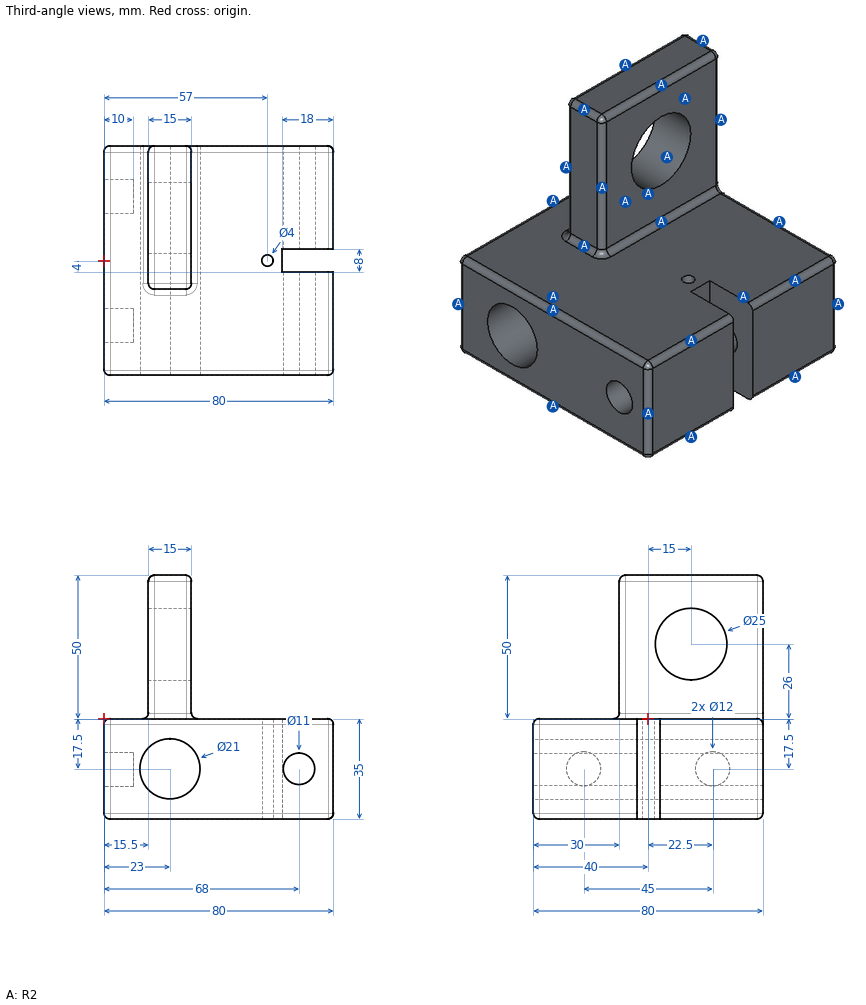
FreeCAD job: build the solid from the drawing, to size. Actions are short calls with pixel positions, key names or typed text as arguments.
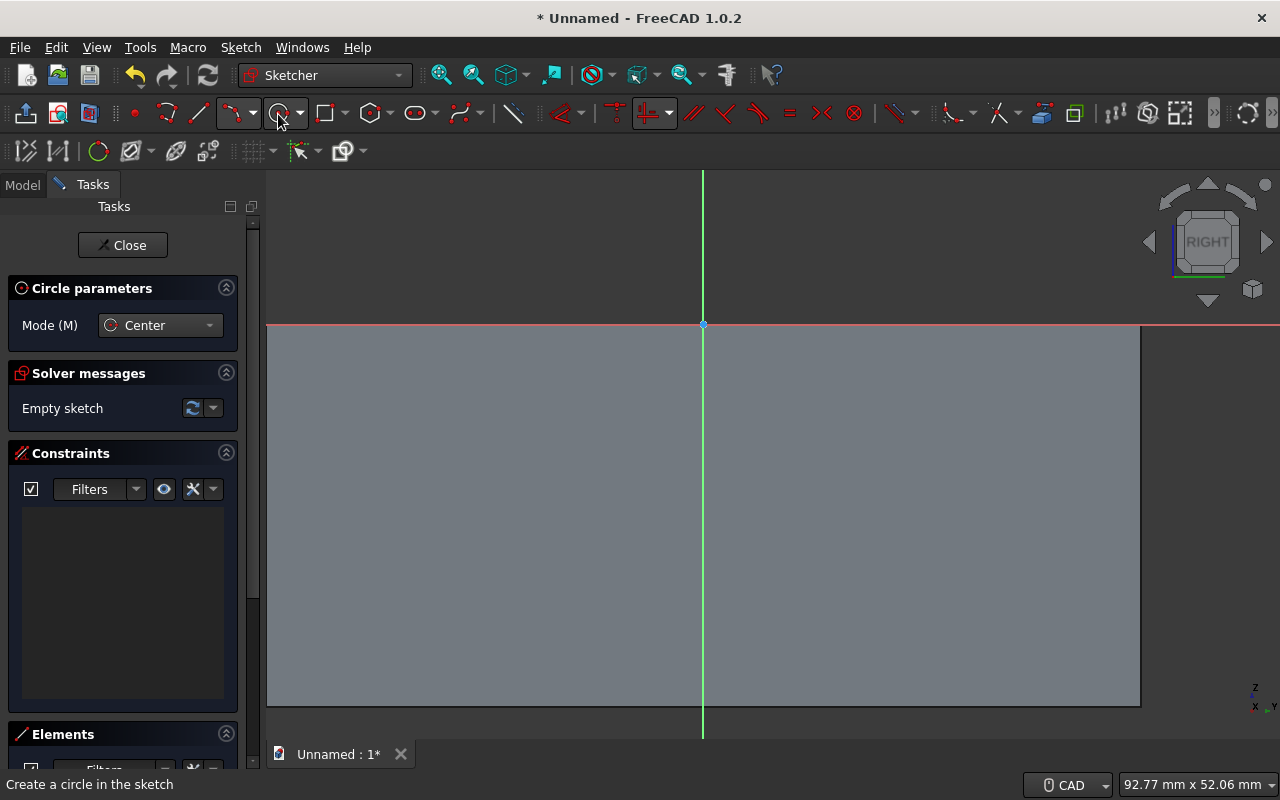
click(949, 516)
click(996, 470)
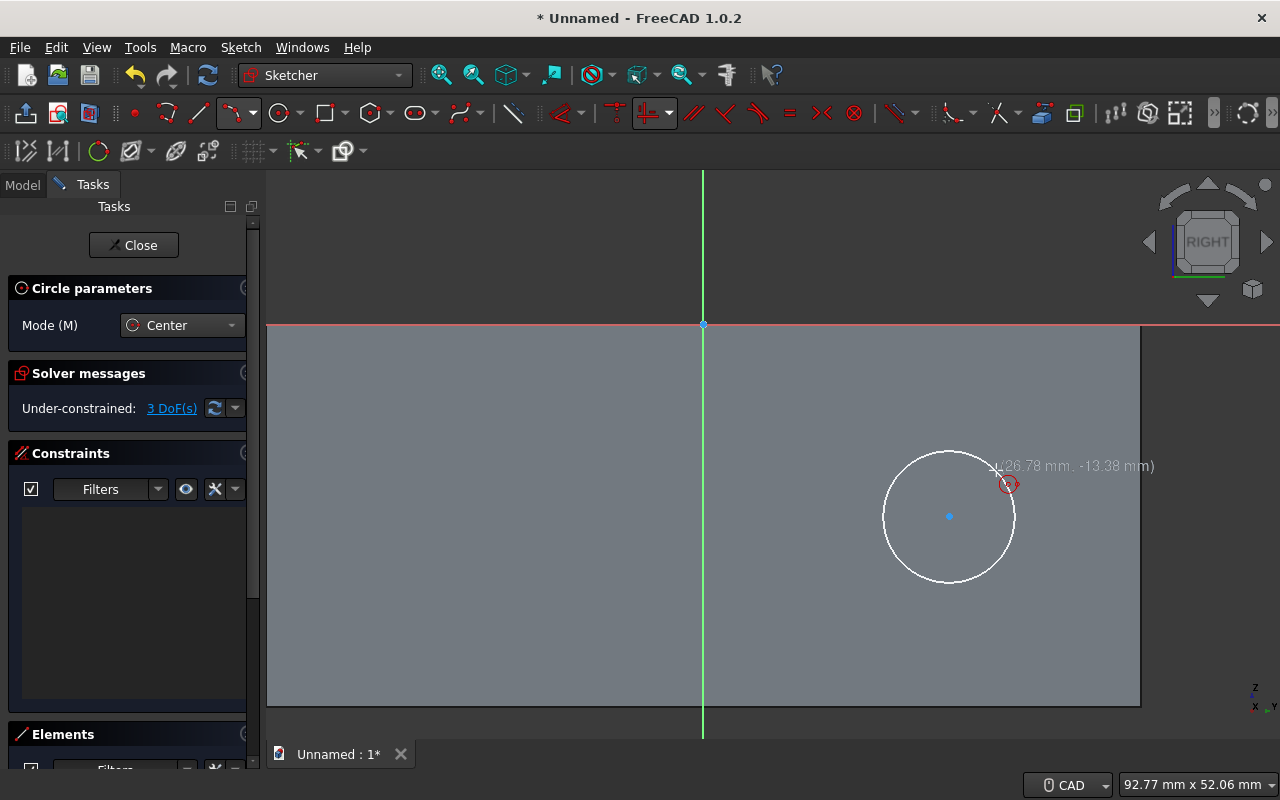
click(457, 516)
click(504, 470)
key(Escape)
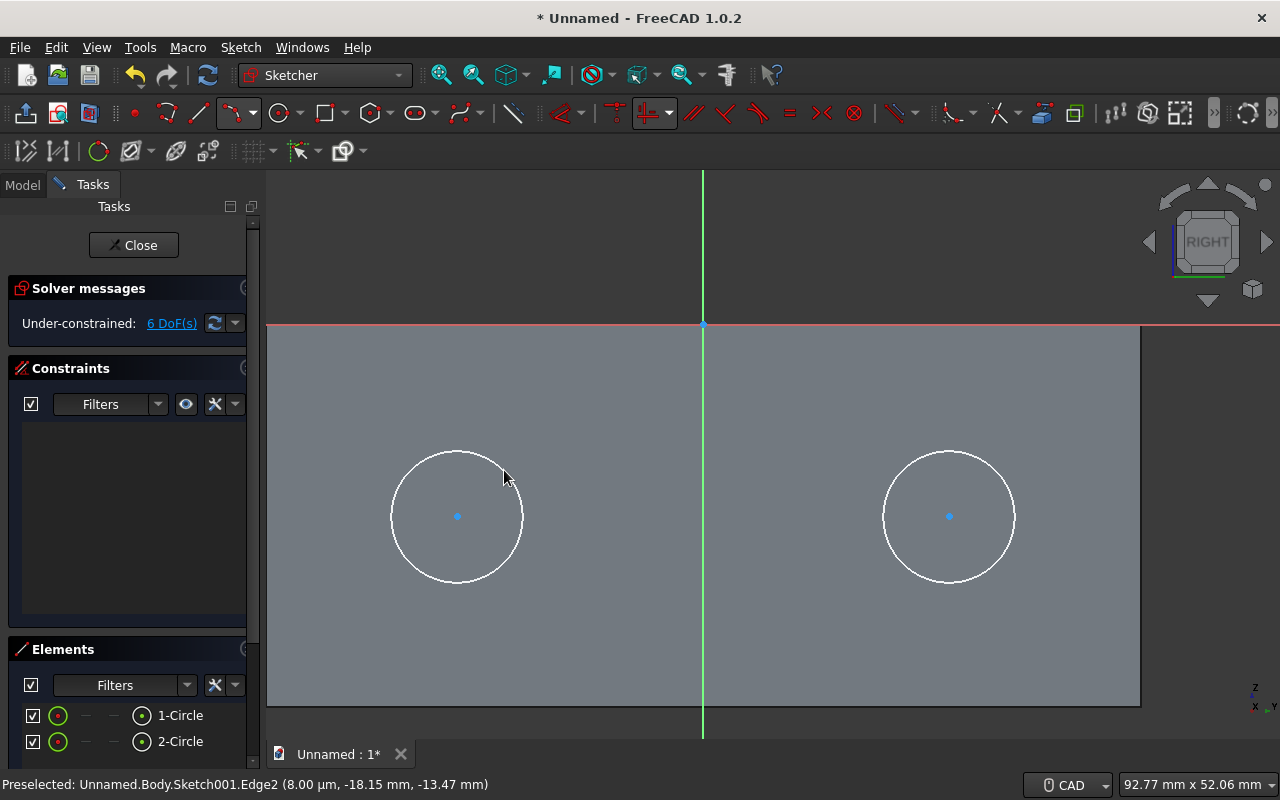
click(995, 470)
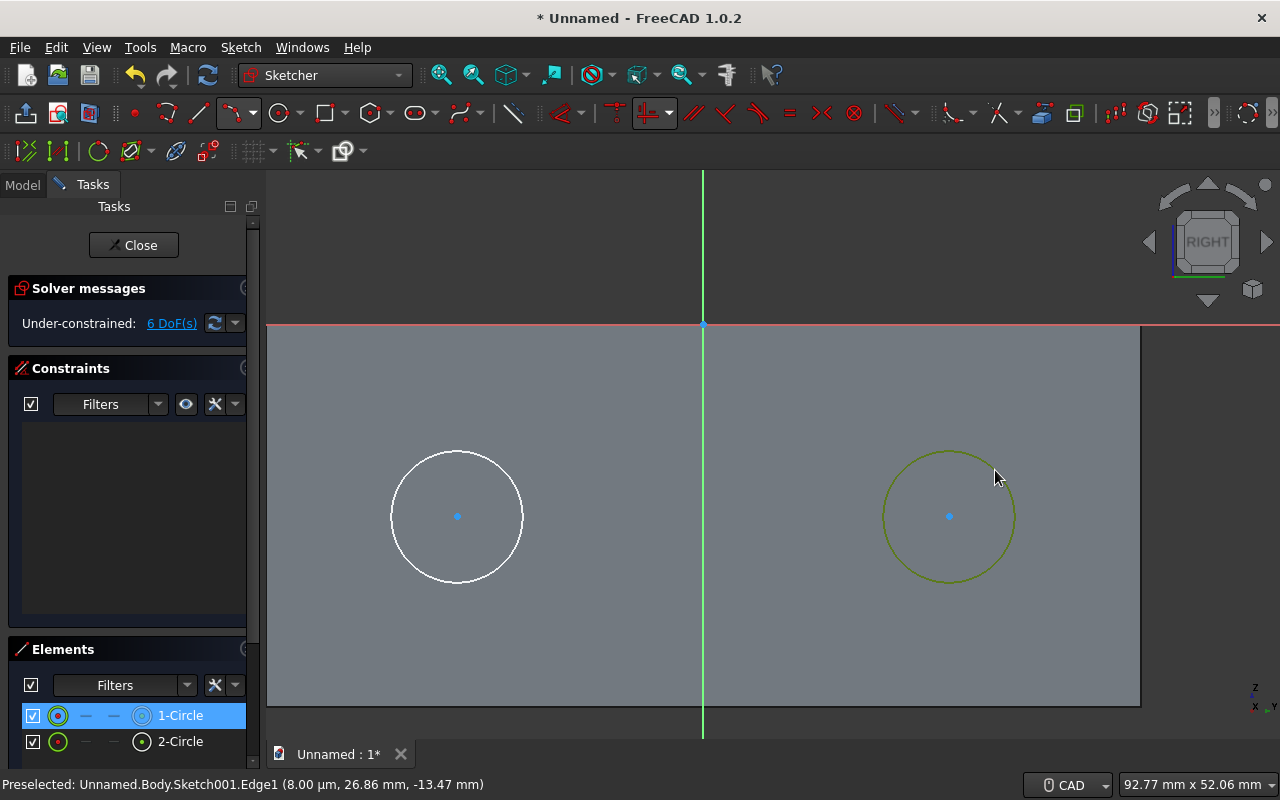
click(503, 470)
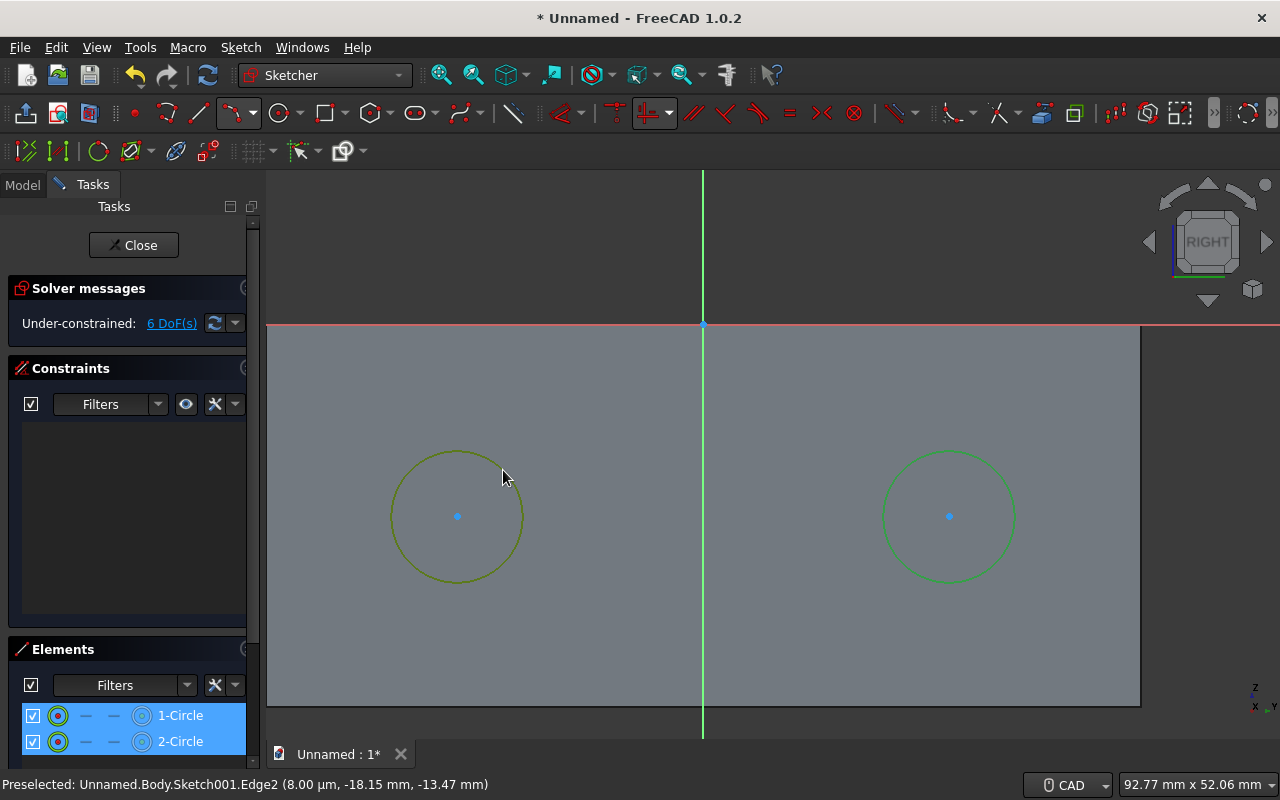
click(790, 114)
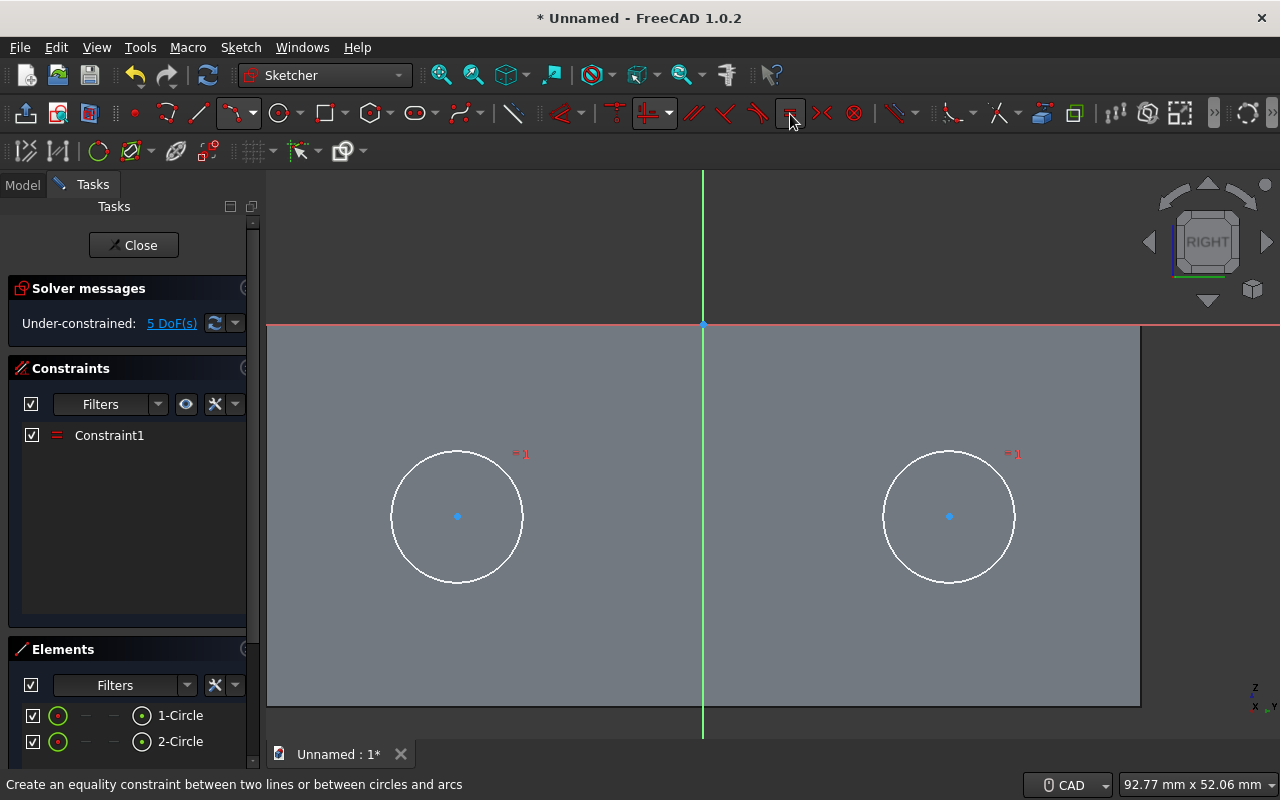
click(949, 517)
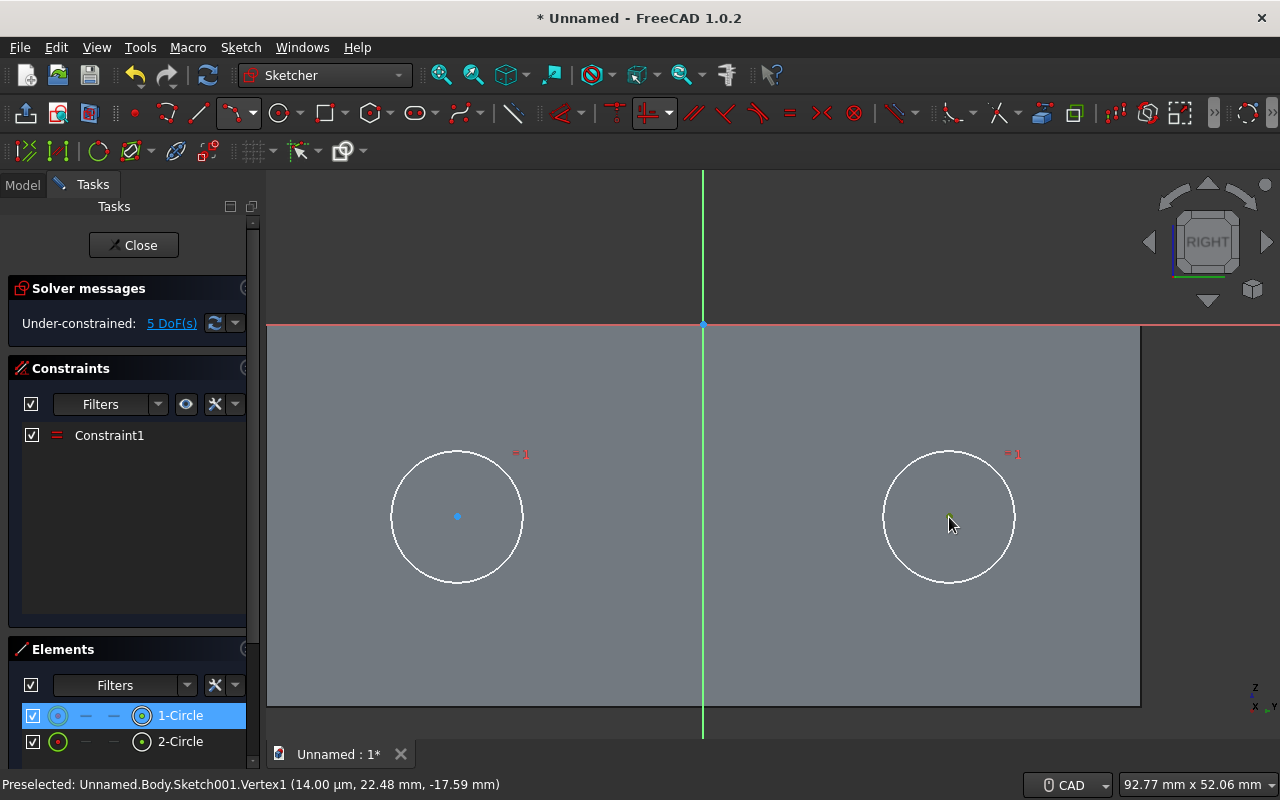
click(457, 517)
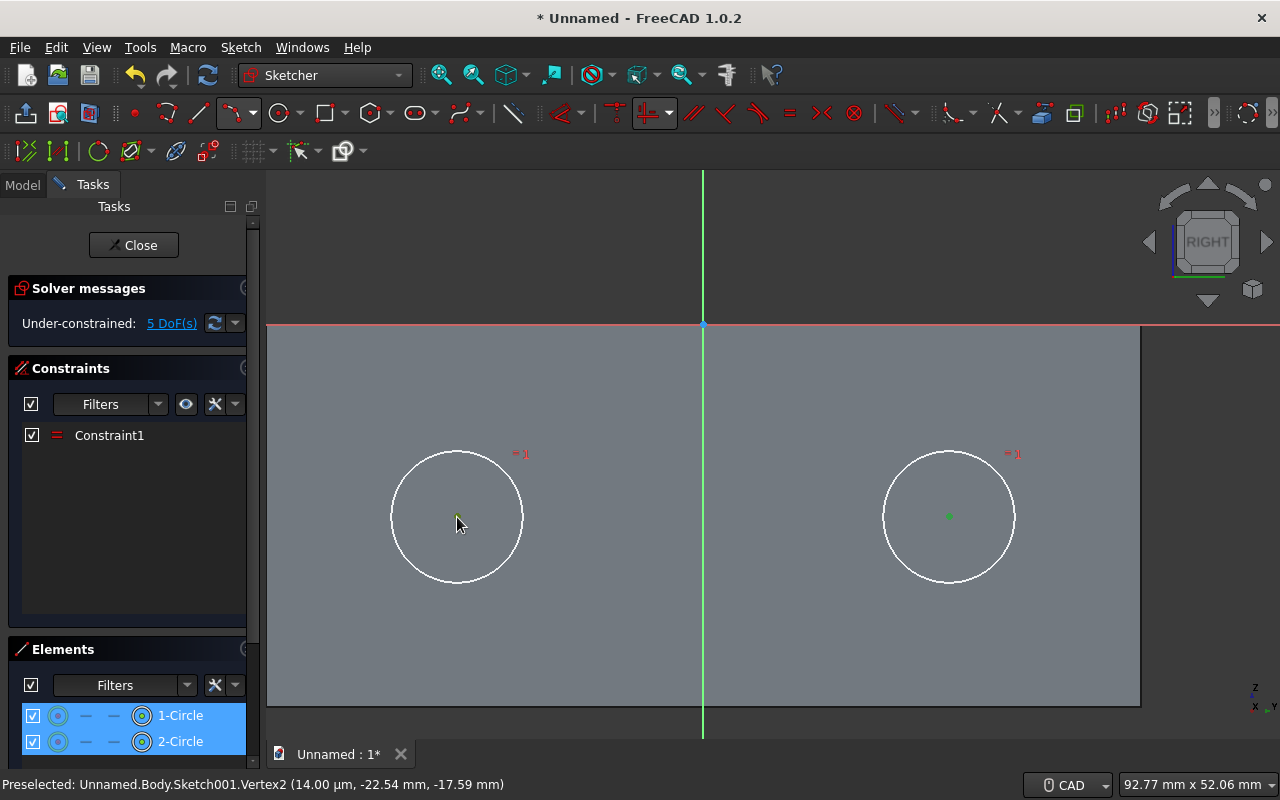
key(h)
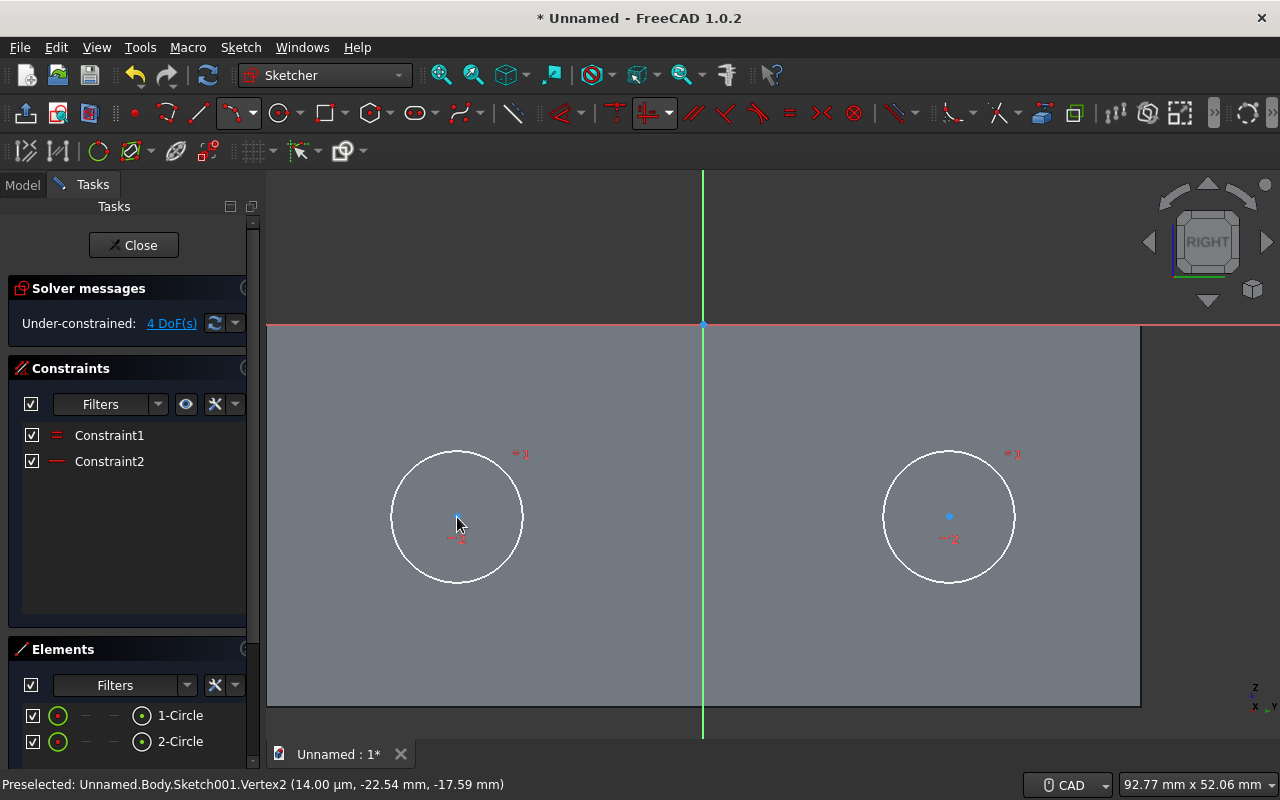
click(560, 114)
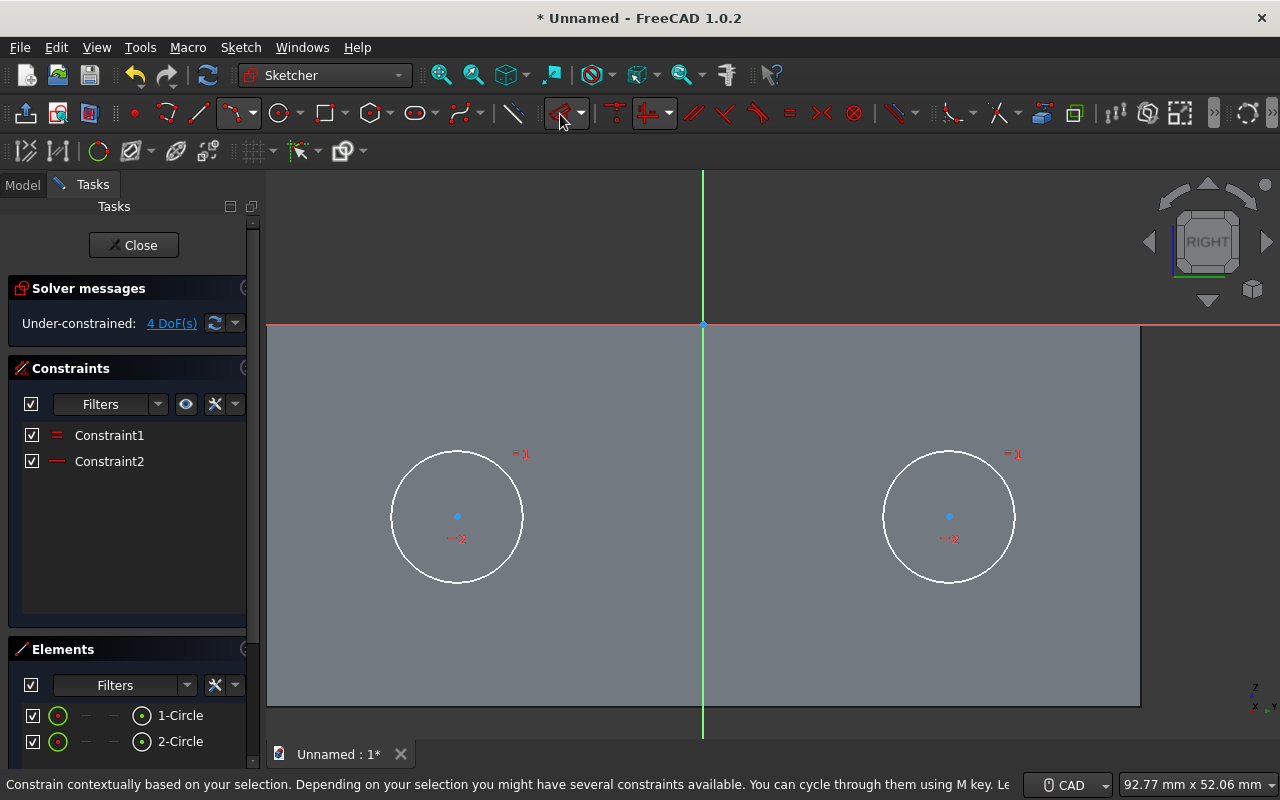
click(995, 470)
click(1017, 447)